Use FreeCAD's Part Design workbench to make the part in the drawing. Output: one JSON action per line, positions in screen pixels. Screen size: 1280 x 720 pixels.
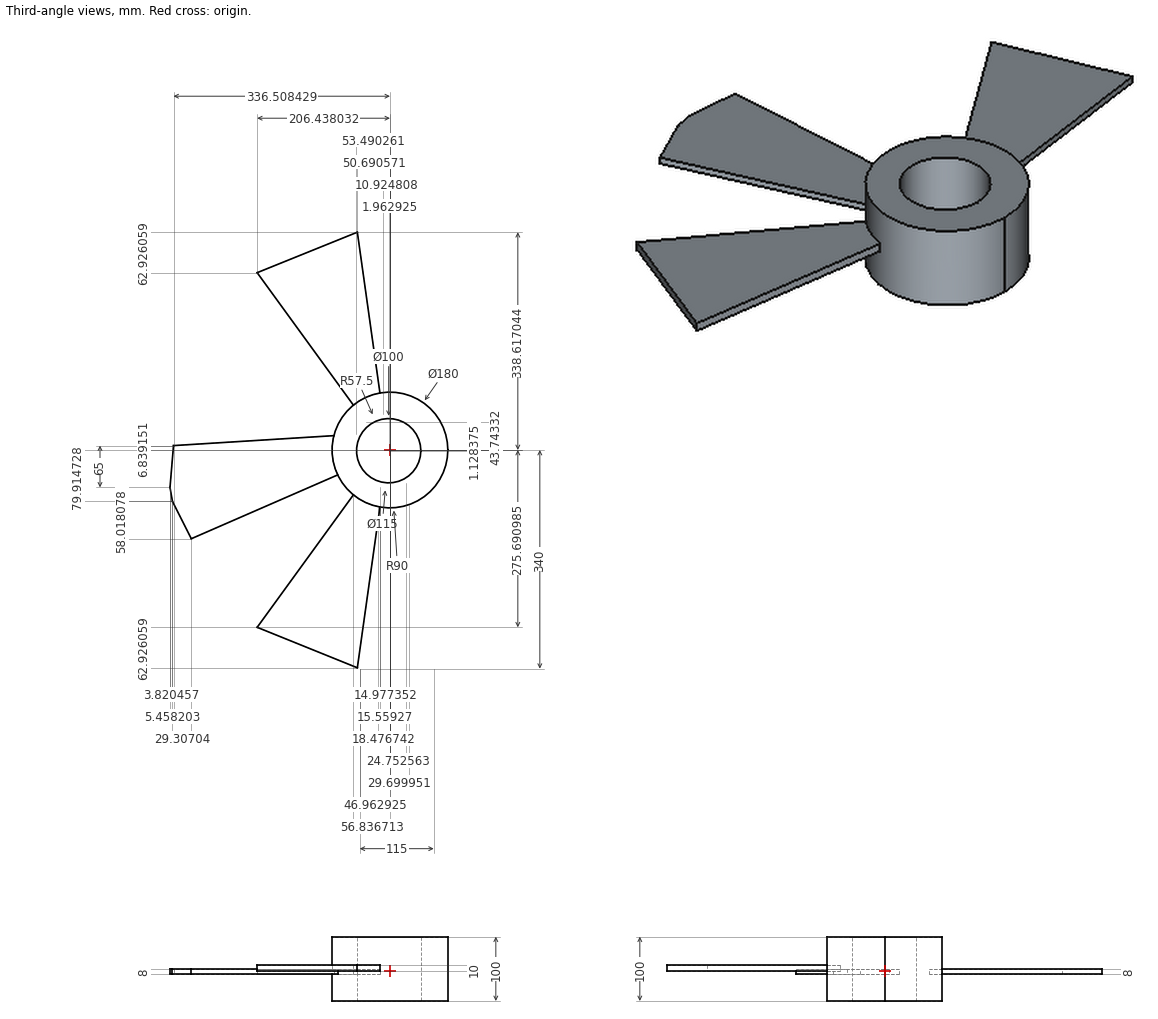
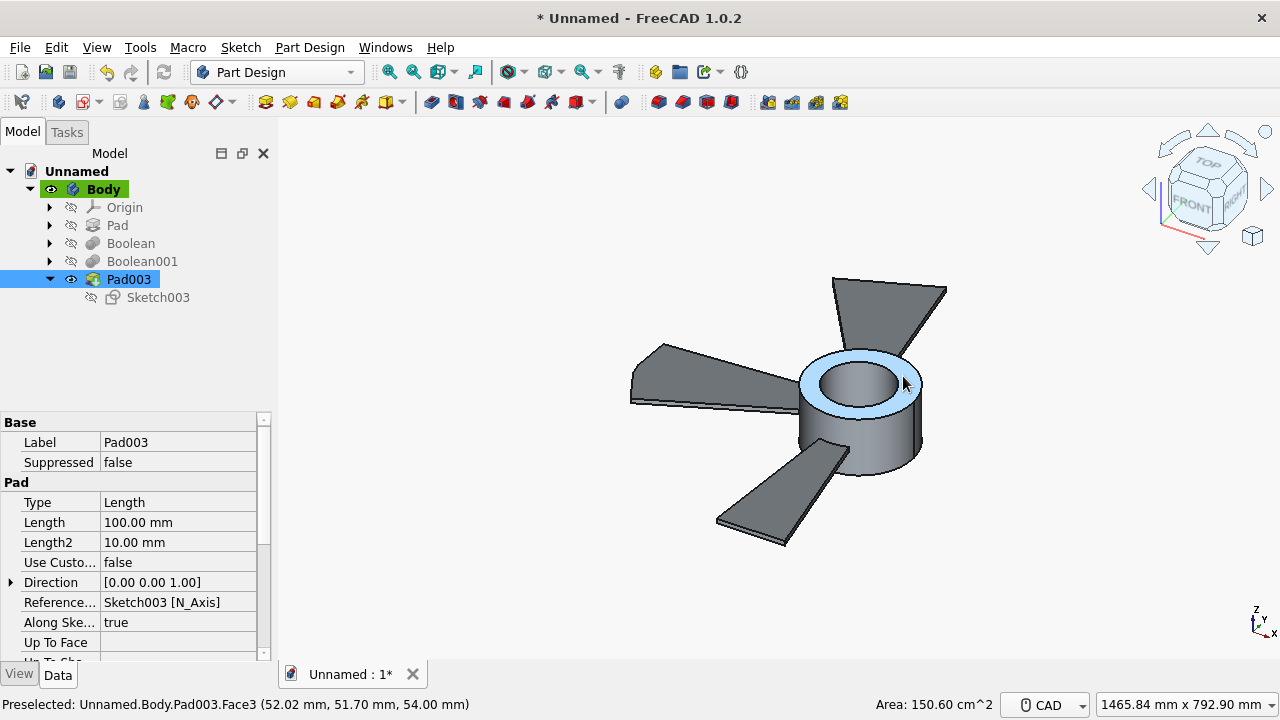
{"action": "left_click", "coordinate": [84, 102]}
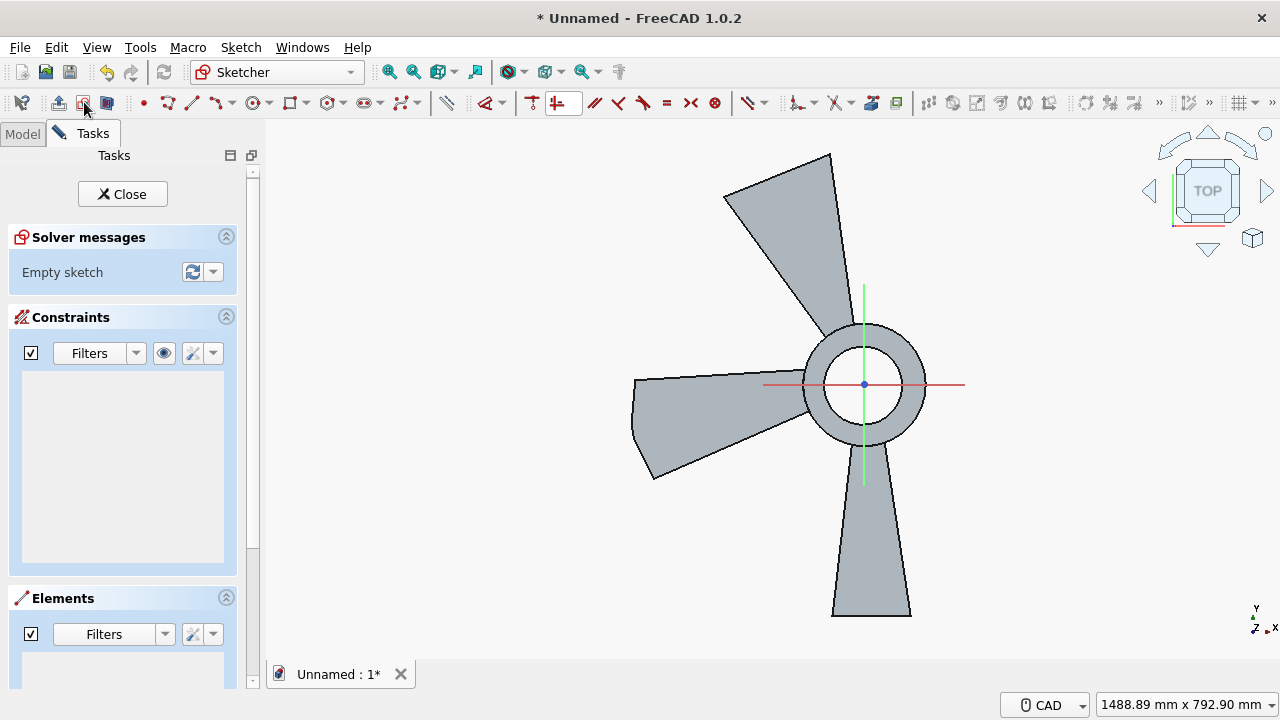
{"action": "scroll", "coordinate": [915, 385], "scroll_direction": "up", "scroll_amount": 7}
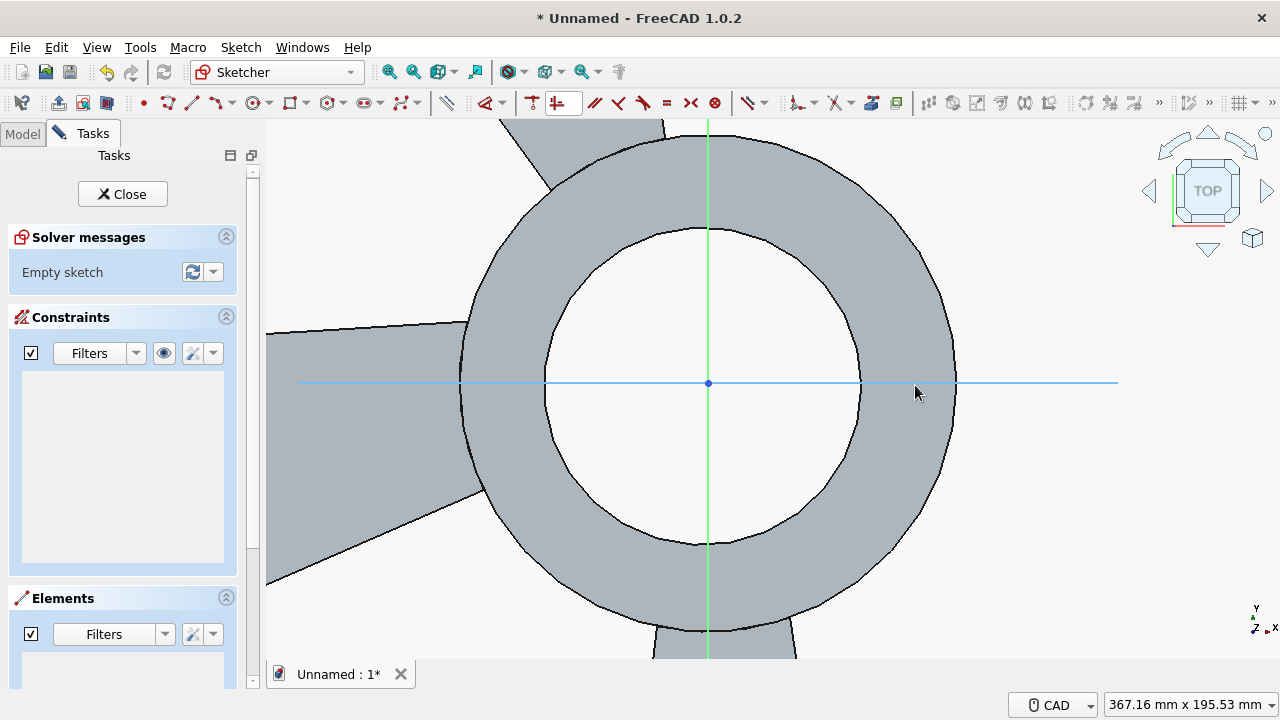
{"action": "left_click", "coordinate": [254, 104]}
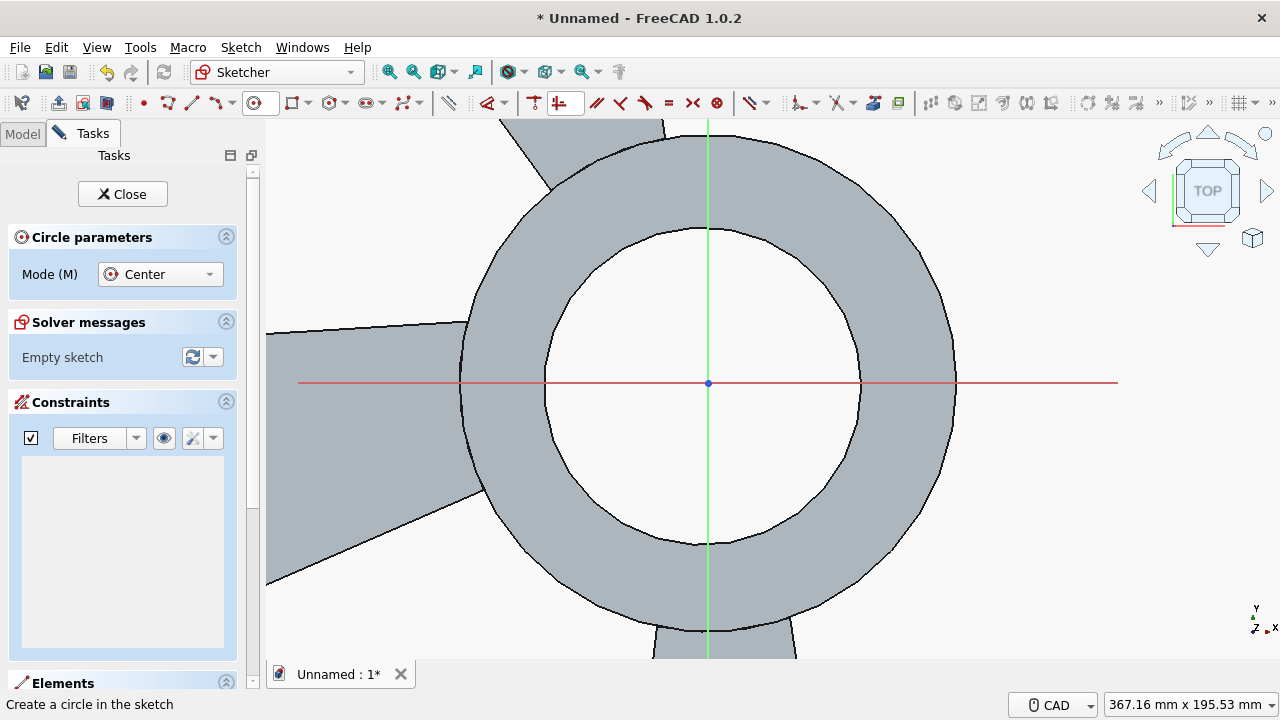
{"action": "scroll", "coordinate": [703, 386], "scroll_direction": "up", "scroll_amount": 9}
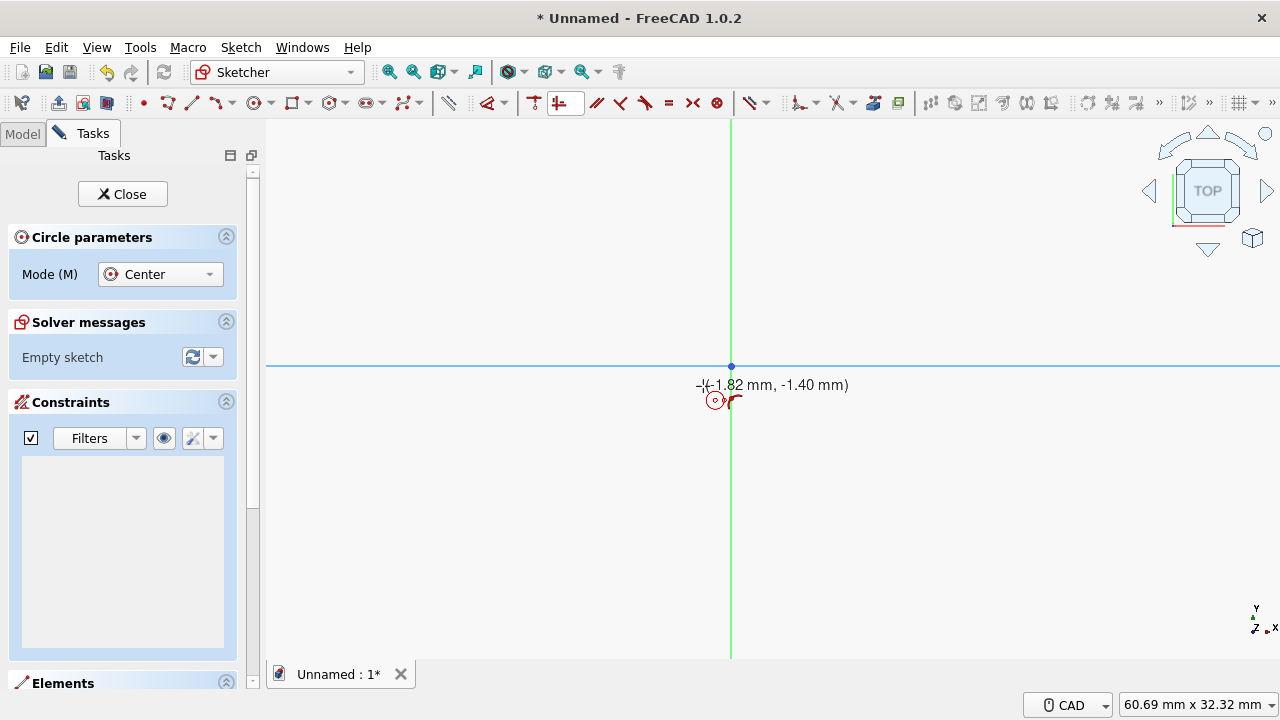
{"action": "left_click", "coordinate": [698, 385]}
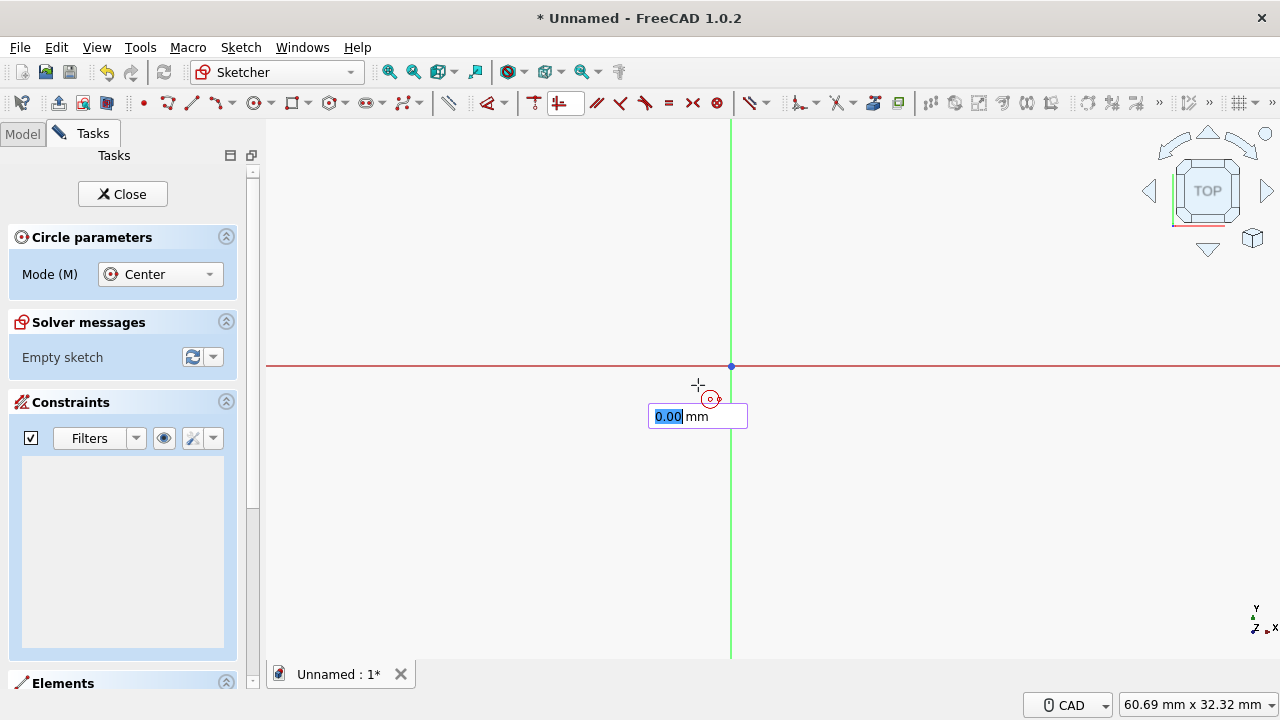
{"action": "scroll", "coordinate": [706, 390], "scroll_direction": "down", "scroll_amount": 9}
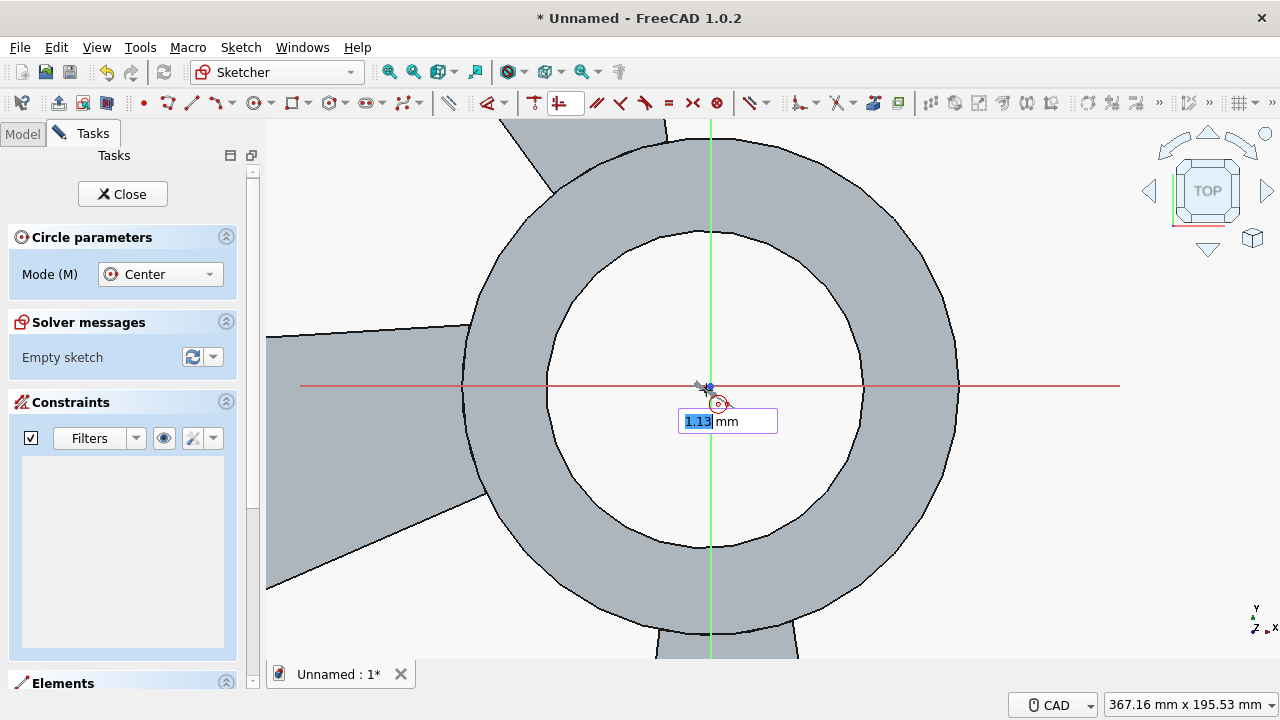
{"action": "left_click", "coordinate": [817, 277]}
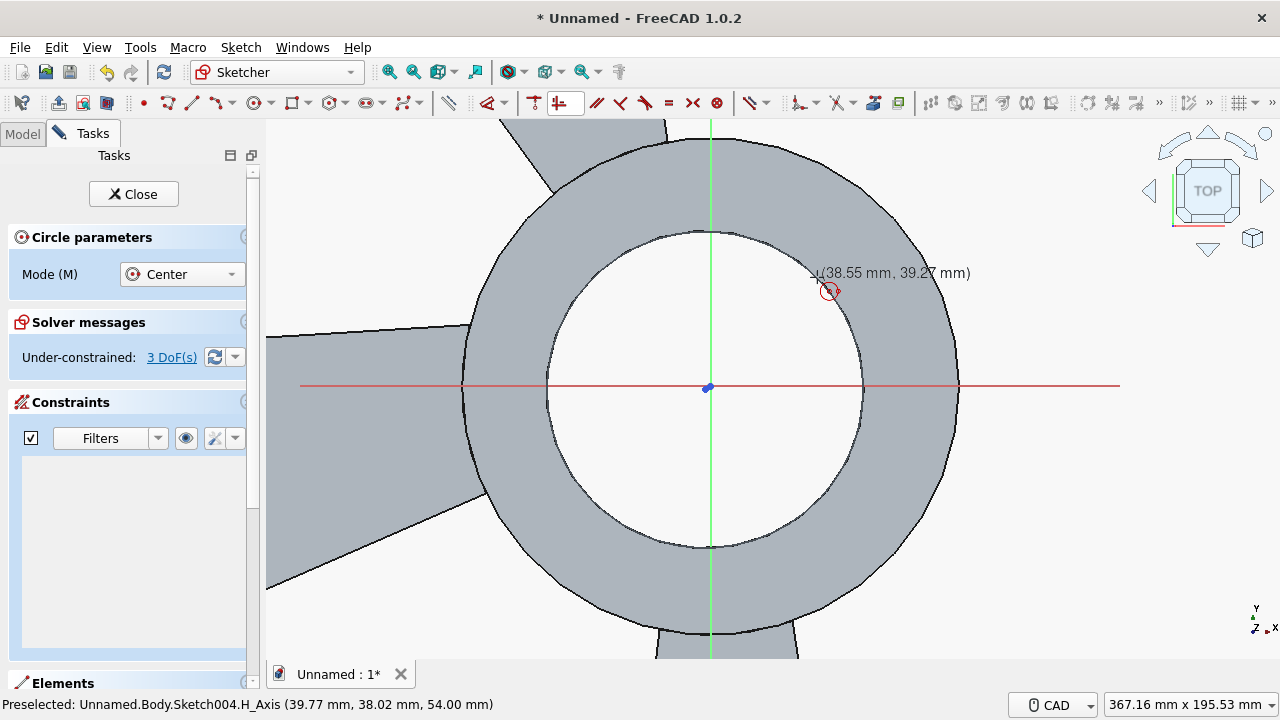
{"action": "scroll", "coordinate": [705, 390], "scroll_direction": "up", "scroll_amount": 9}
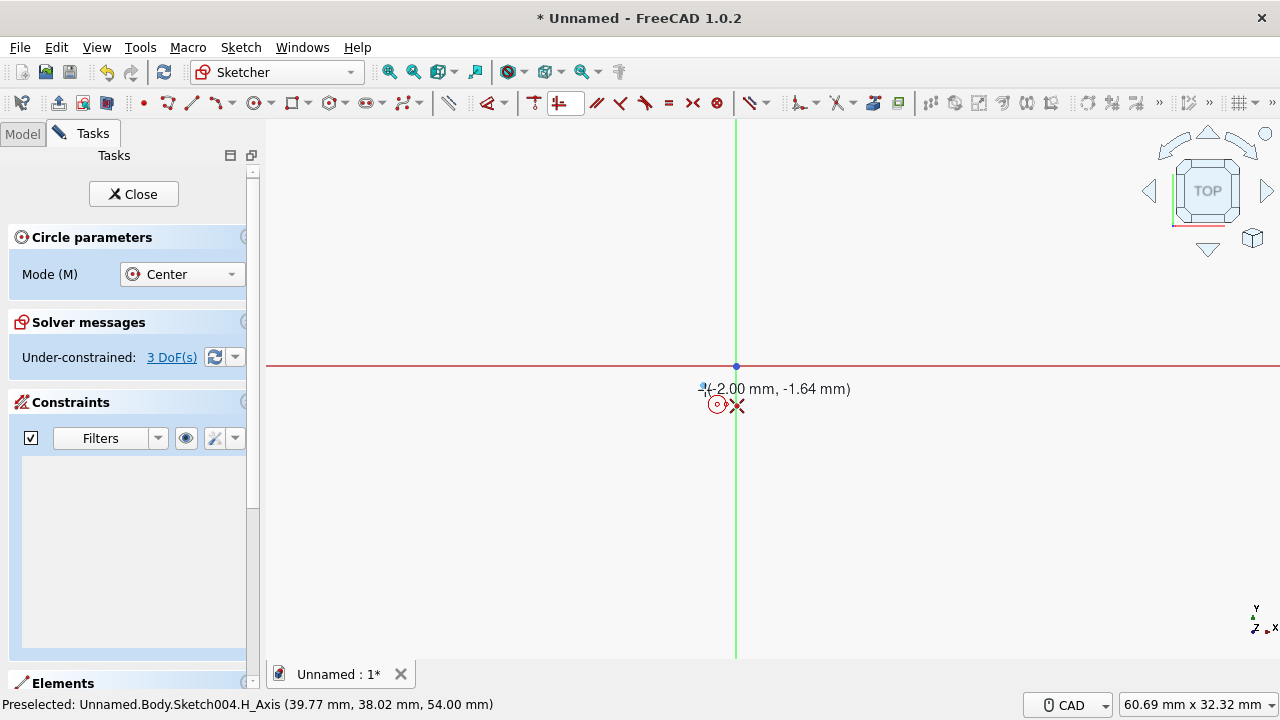
{"action": "left_click", "coordinate": [703, 386]}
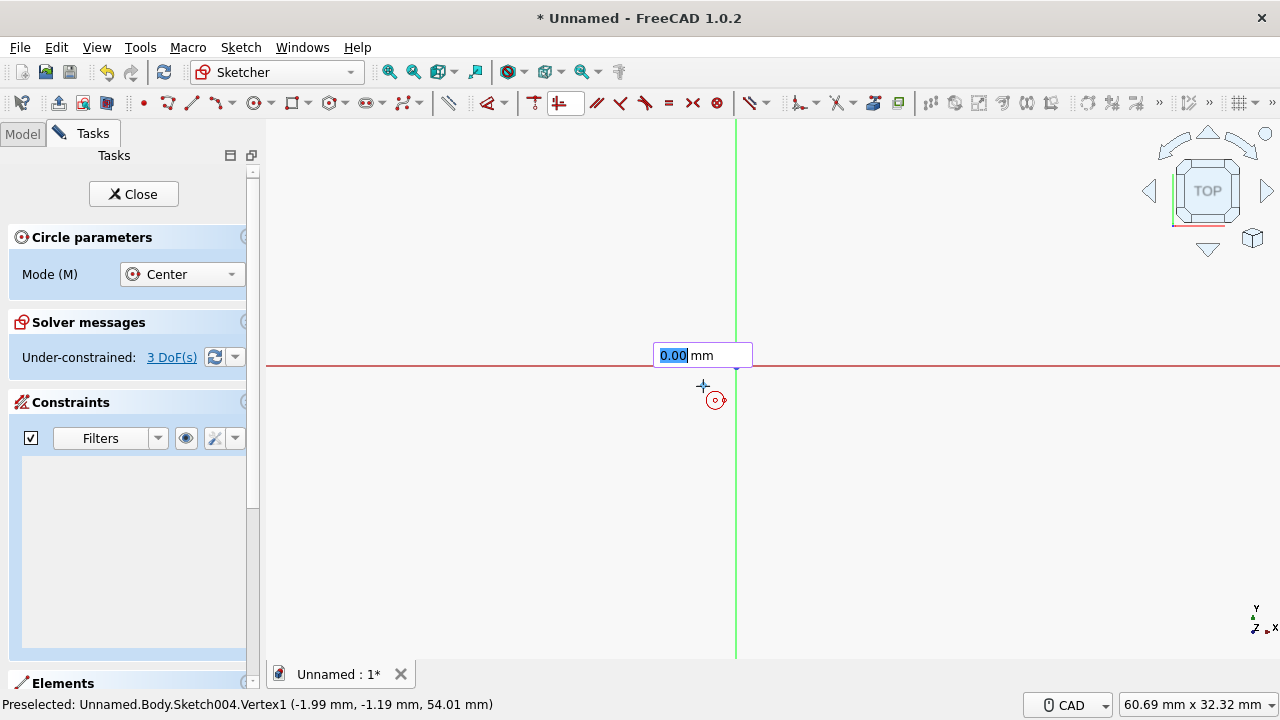
{"action": "scroll", "coordinate": [705, 390], "scroll_direction": "down", "scroll_amount": 9}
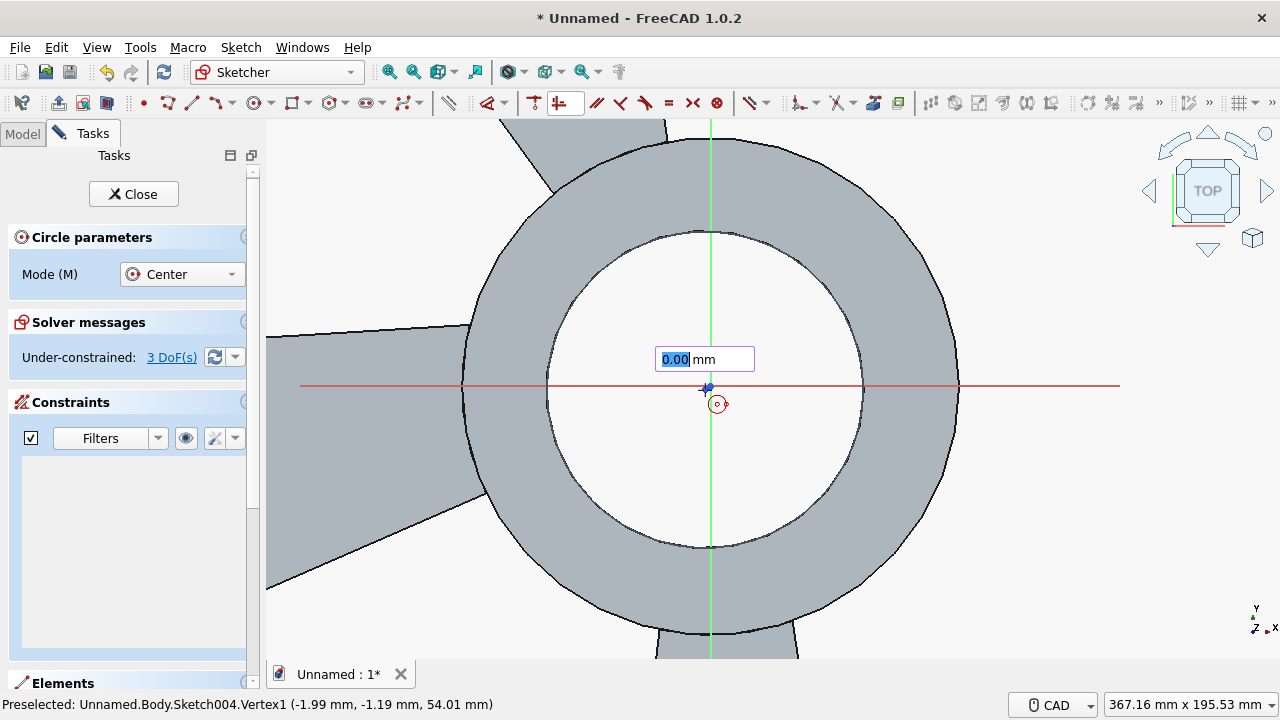
{"action": "left_click", "coordinate": [803, 292]}
{"action": "key", "text": "Escape"}